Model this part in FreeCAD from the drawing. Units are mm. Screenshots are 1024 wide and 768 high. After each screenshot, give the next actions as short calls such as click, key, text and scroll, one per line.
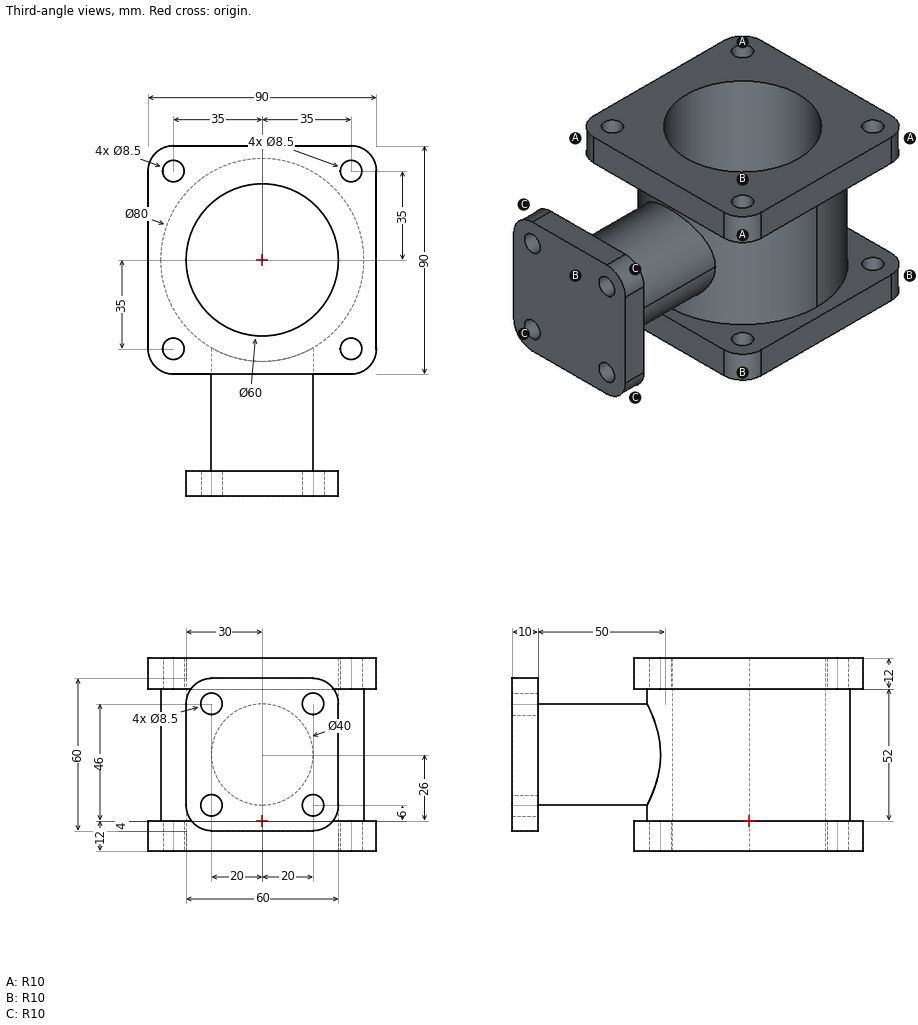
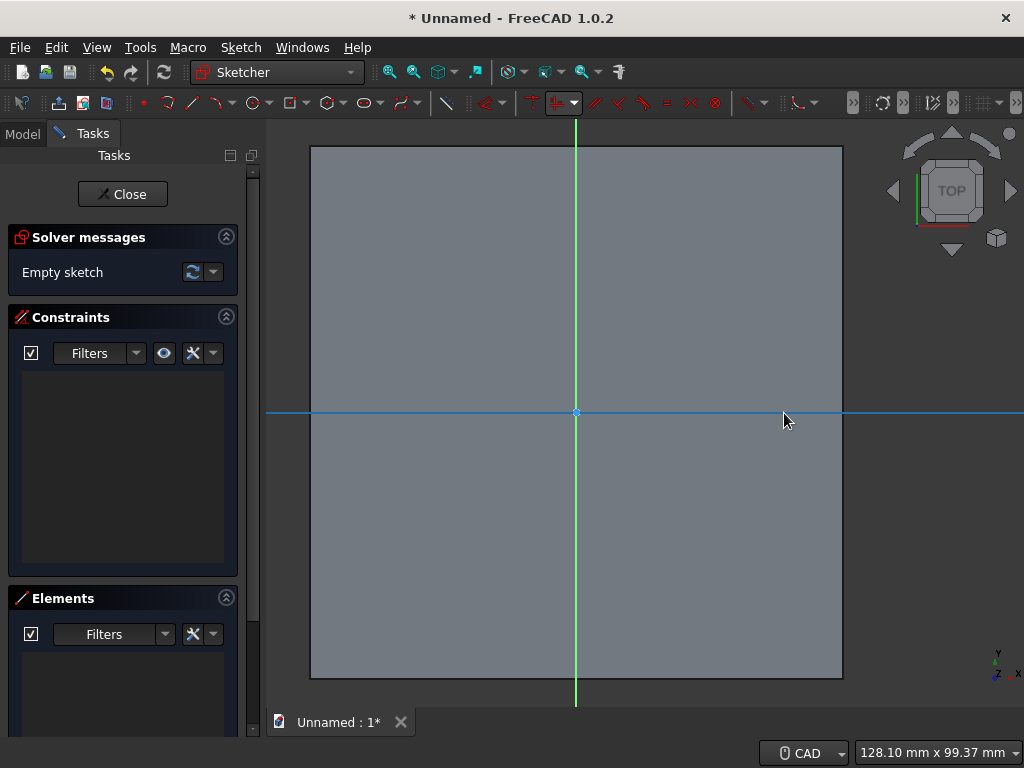
click(254, 104)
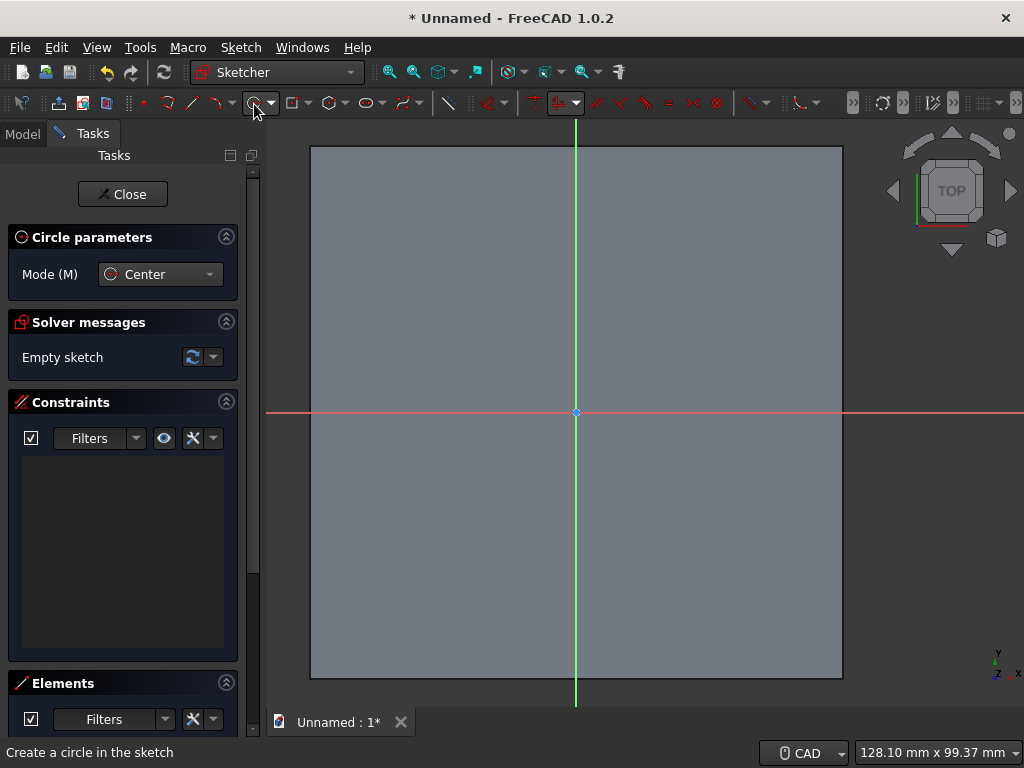
click(576, 413)
click(702, 287)
key(Escape)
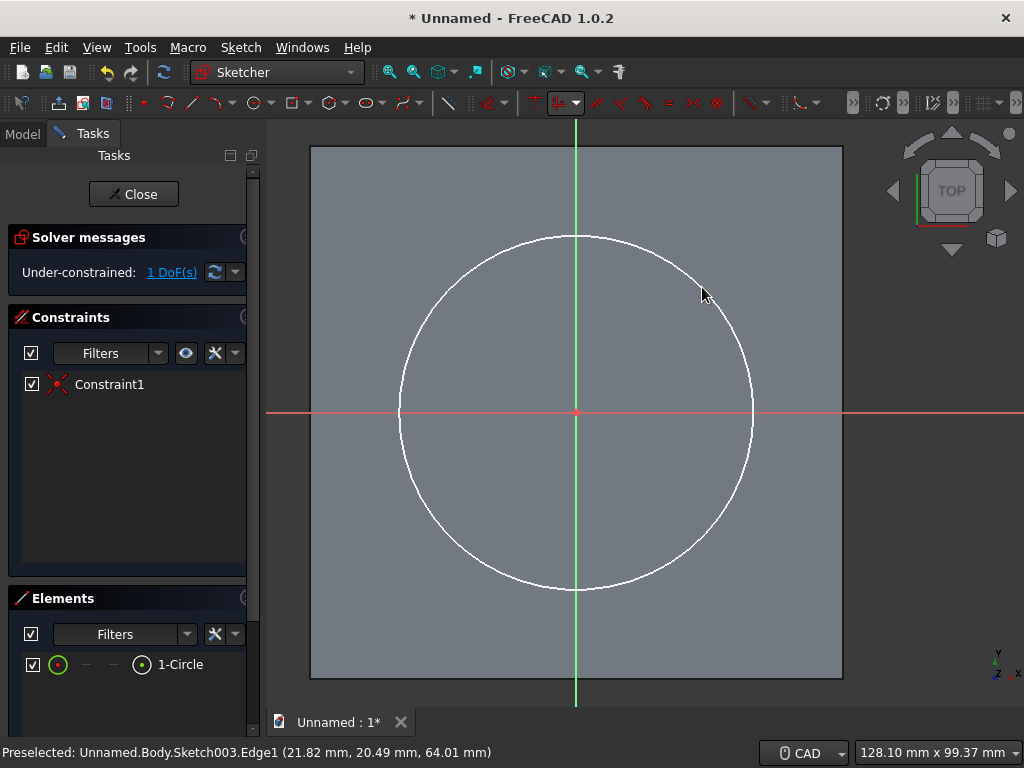
key(d)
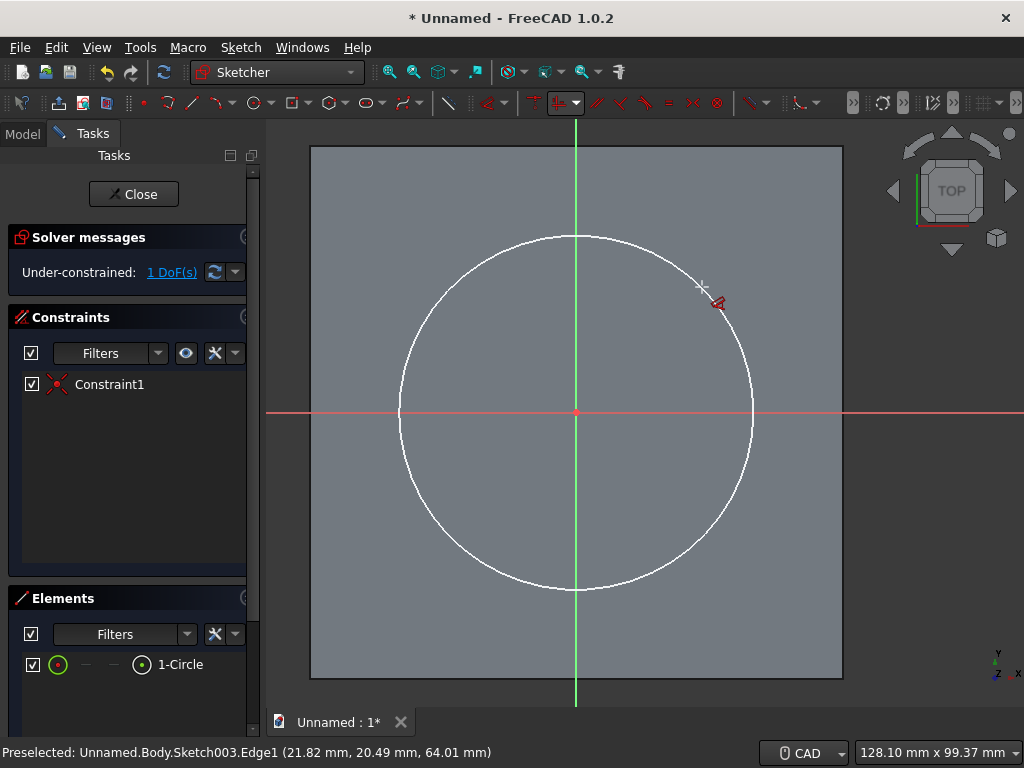
click(701, 287)
click(724, 264)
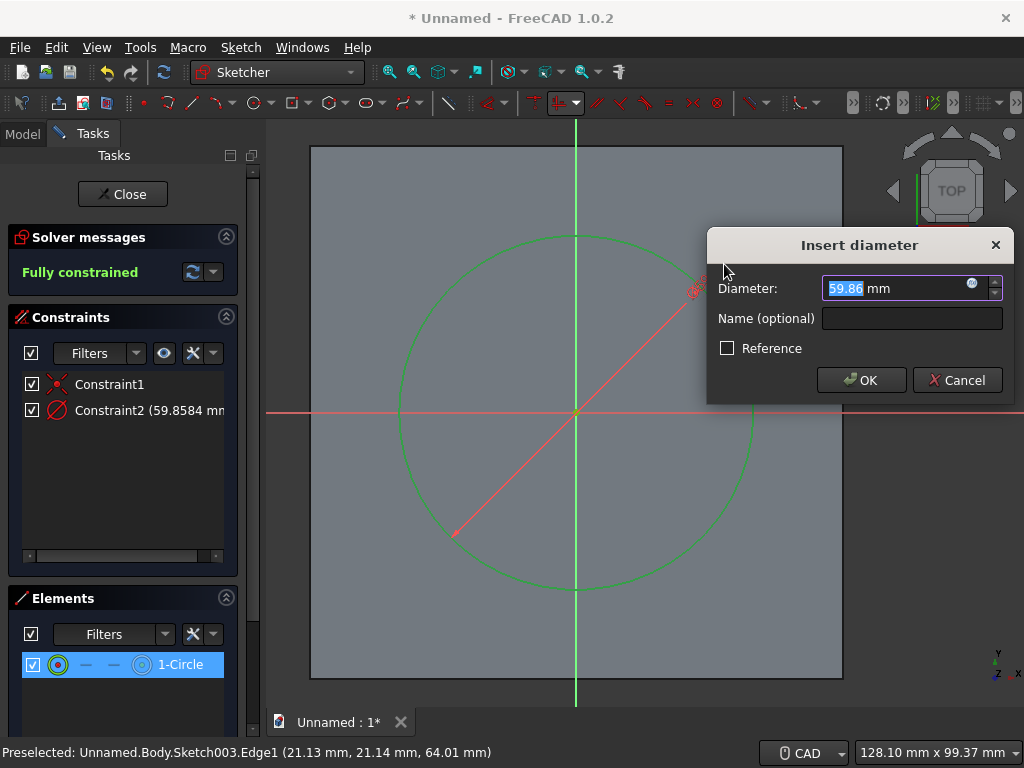
text(60)
key(Return)
key(Escape)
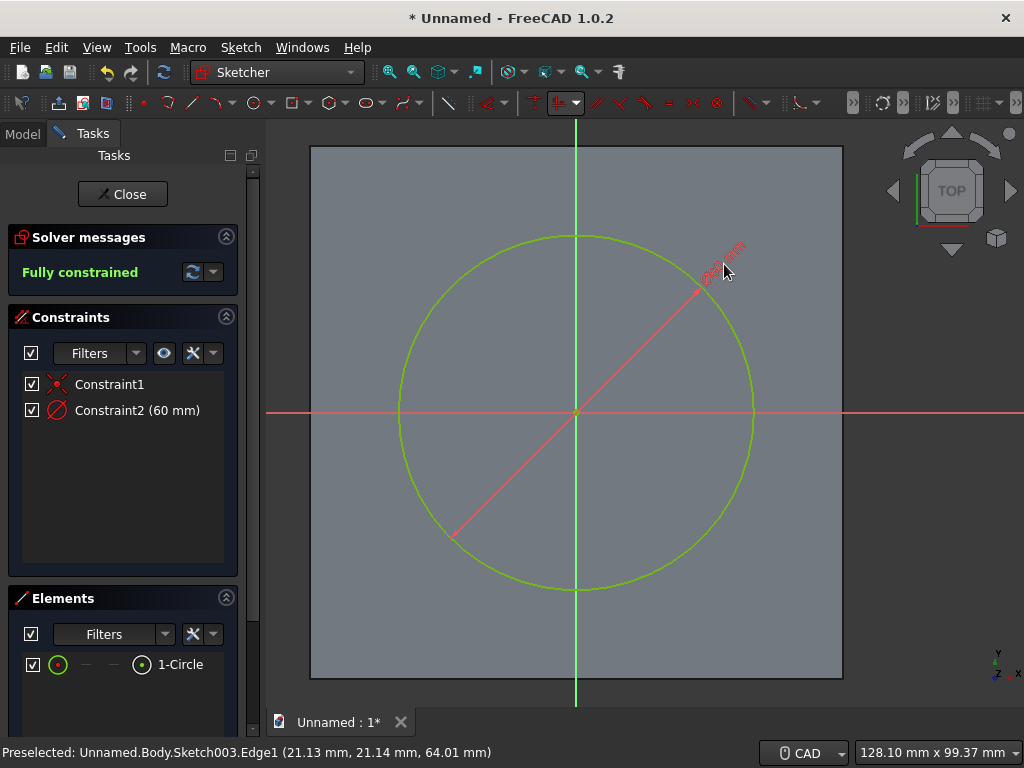
click(123, 194)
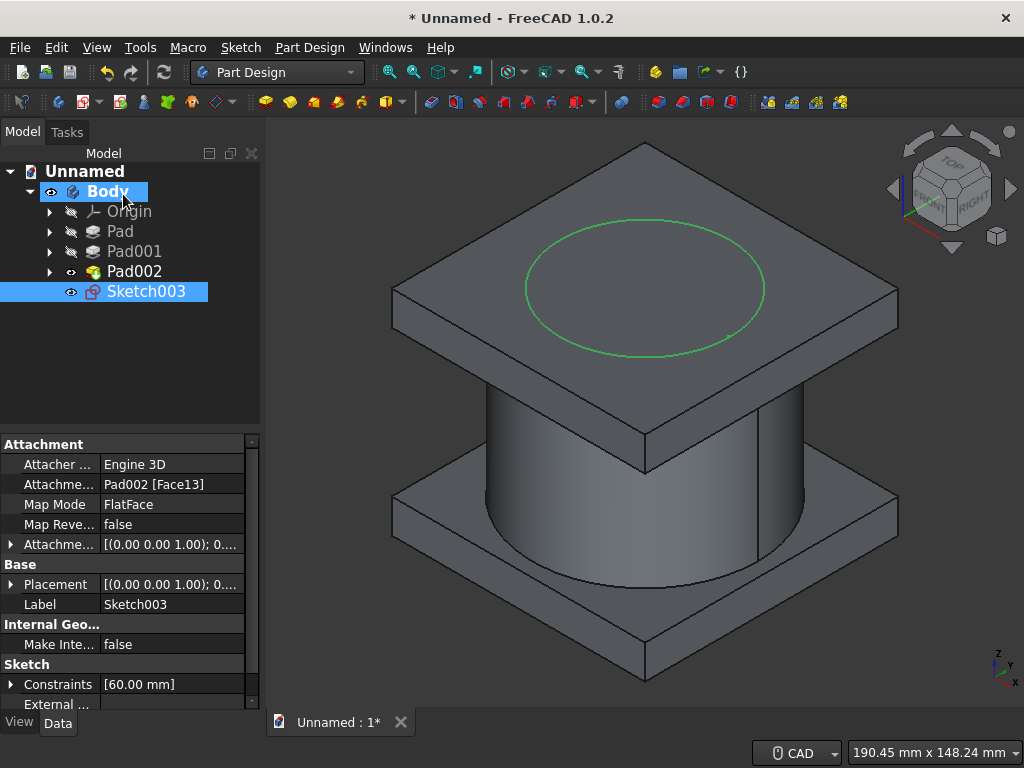
click(432, 102)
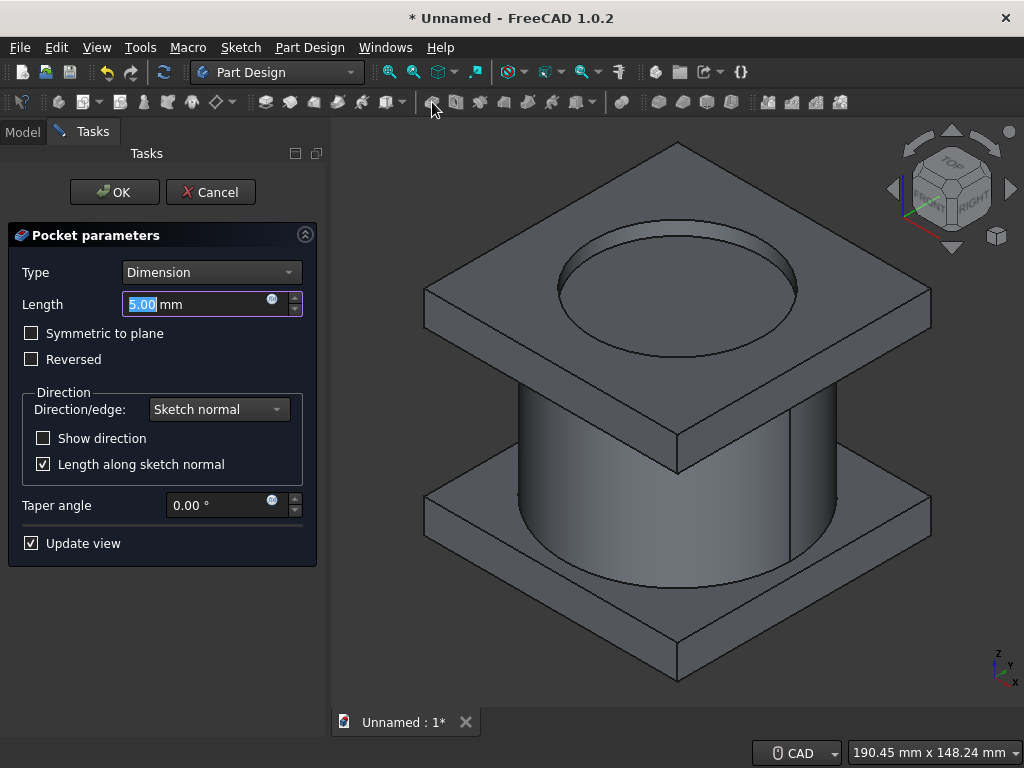
click(212, 272)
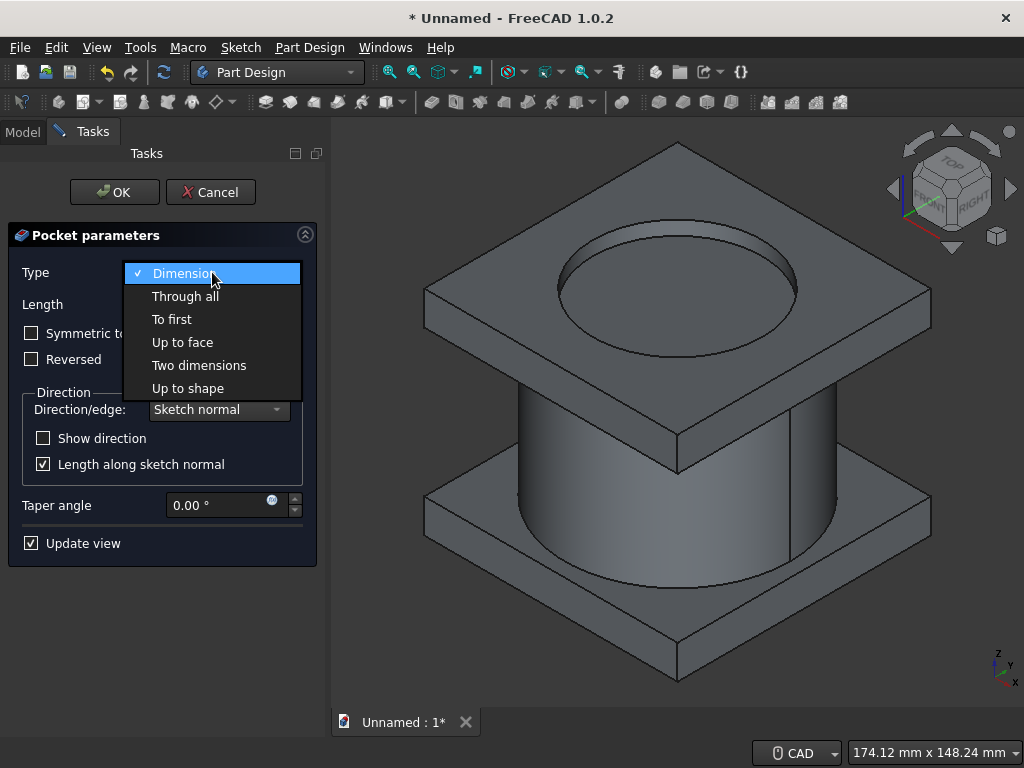
click(212, 296)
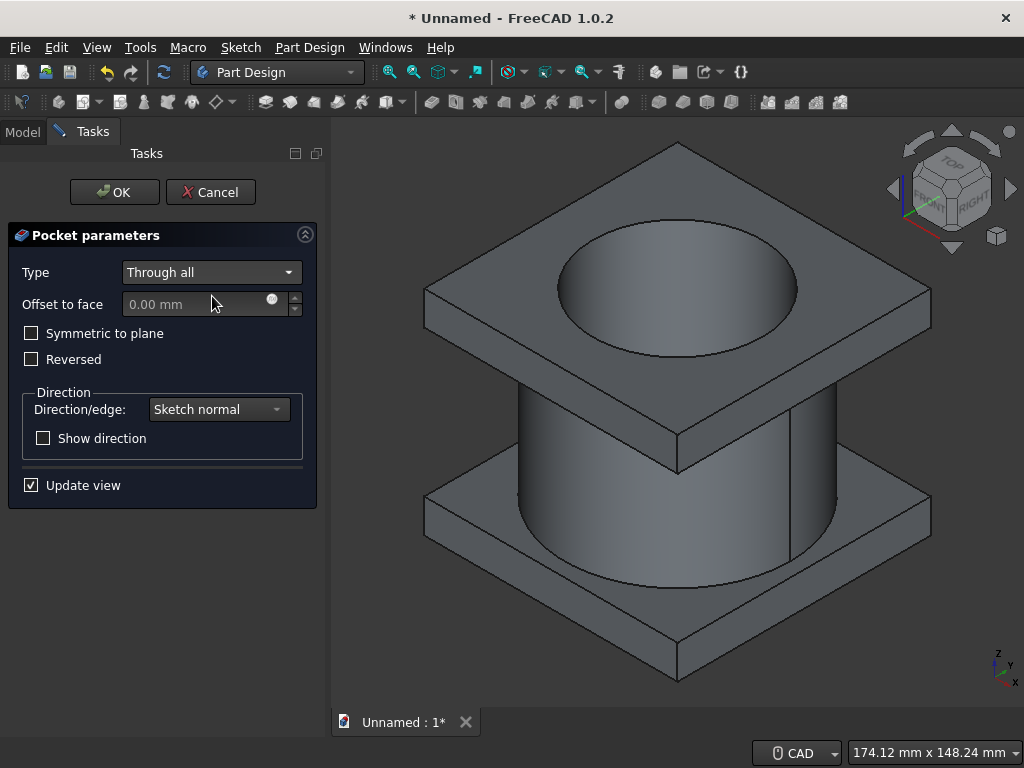
click(115, 192)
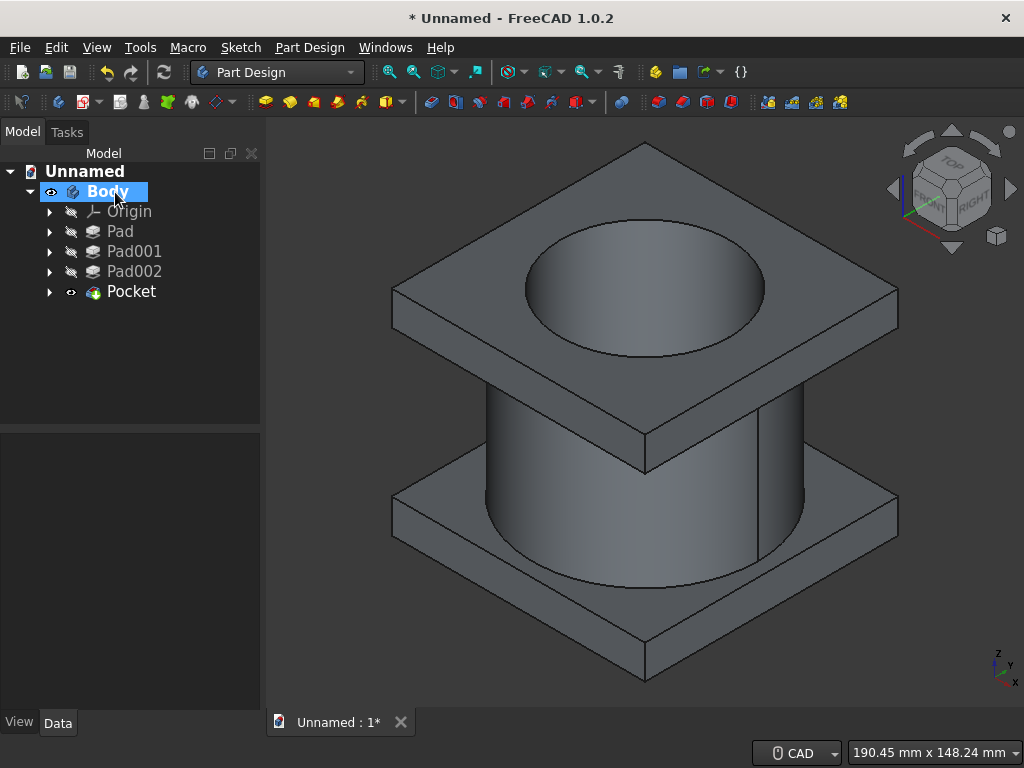
click(645, 453)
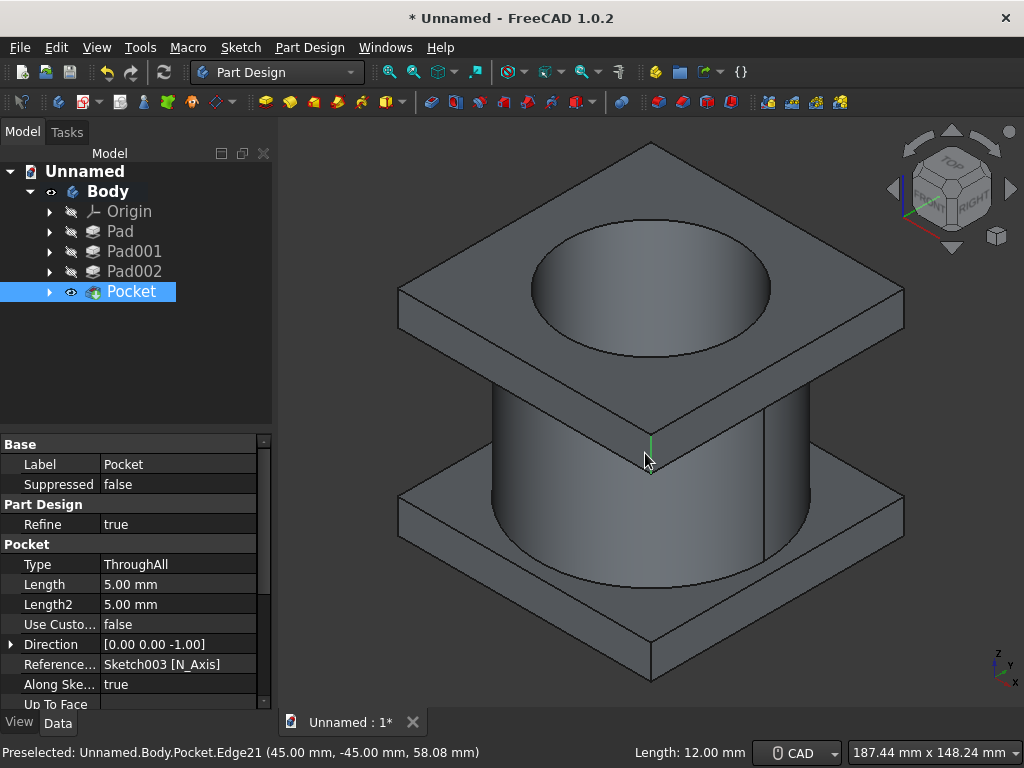
key(2)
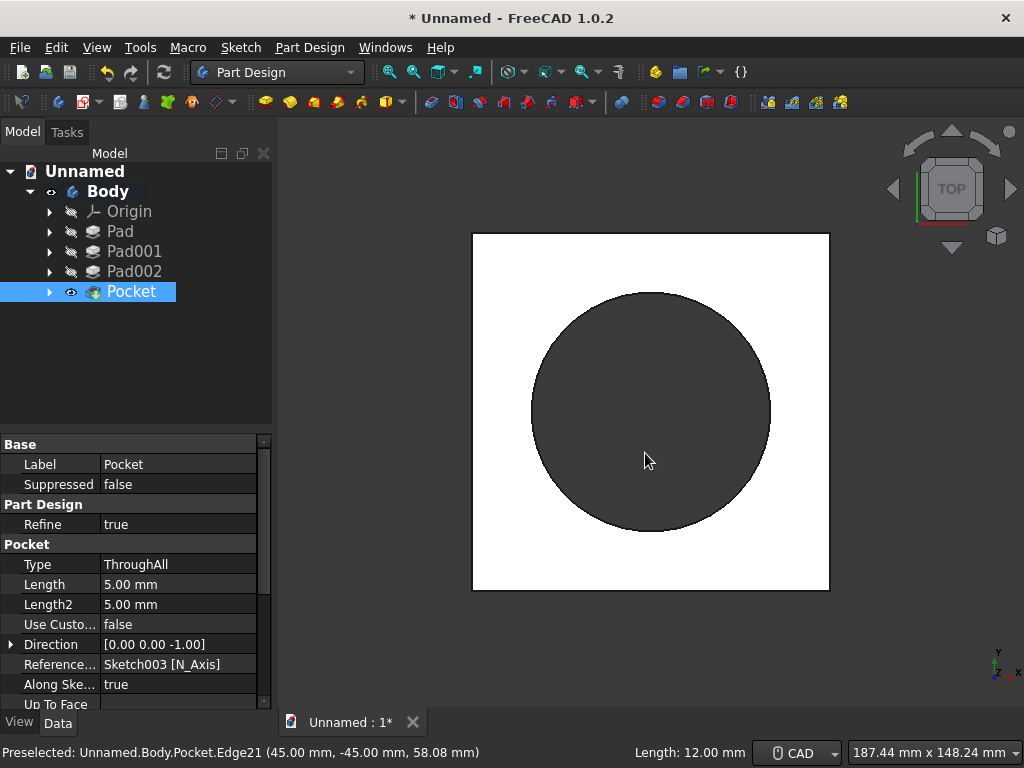
key(0)